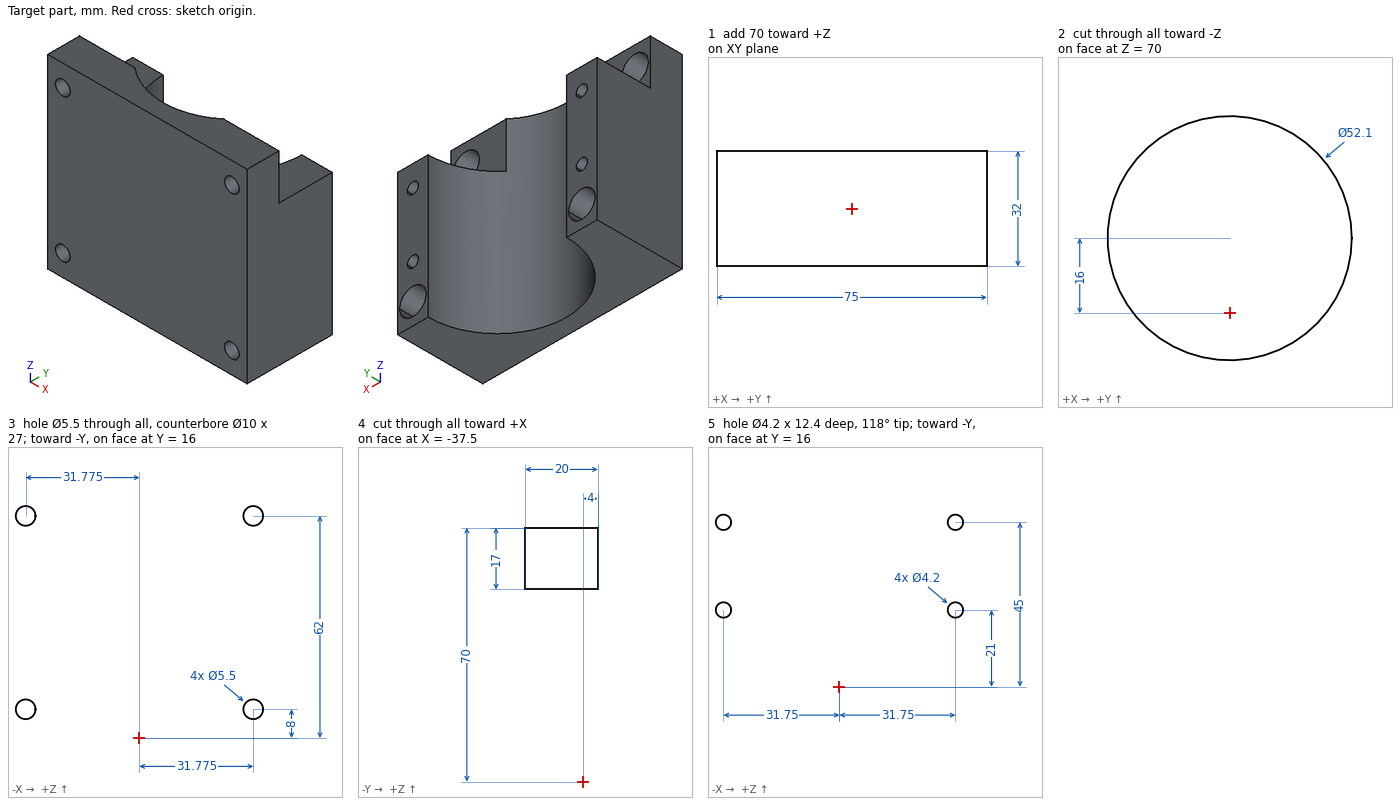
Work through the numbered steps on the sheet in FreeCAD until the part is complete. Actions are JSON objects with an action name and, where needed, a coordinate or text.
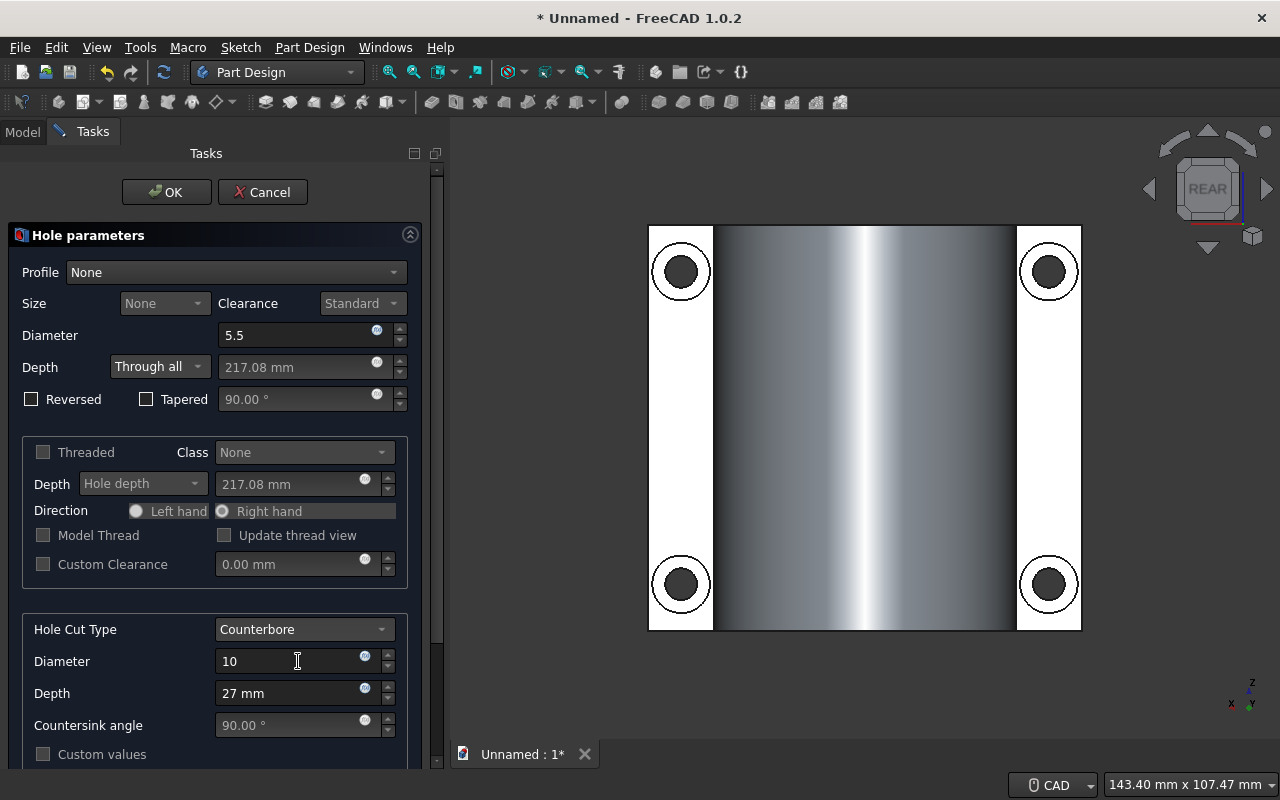
{"action": "left_click", "coordinate": [167, 192]}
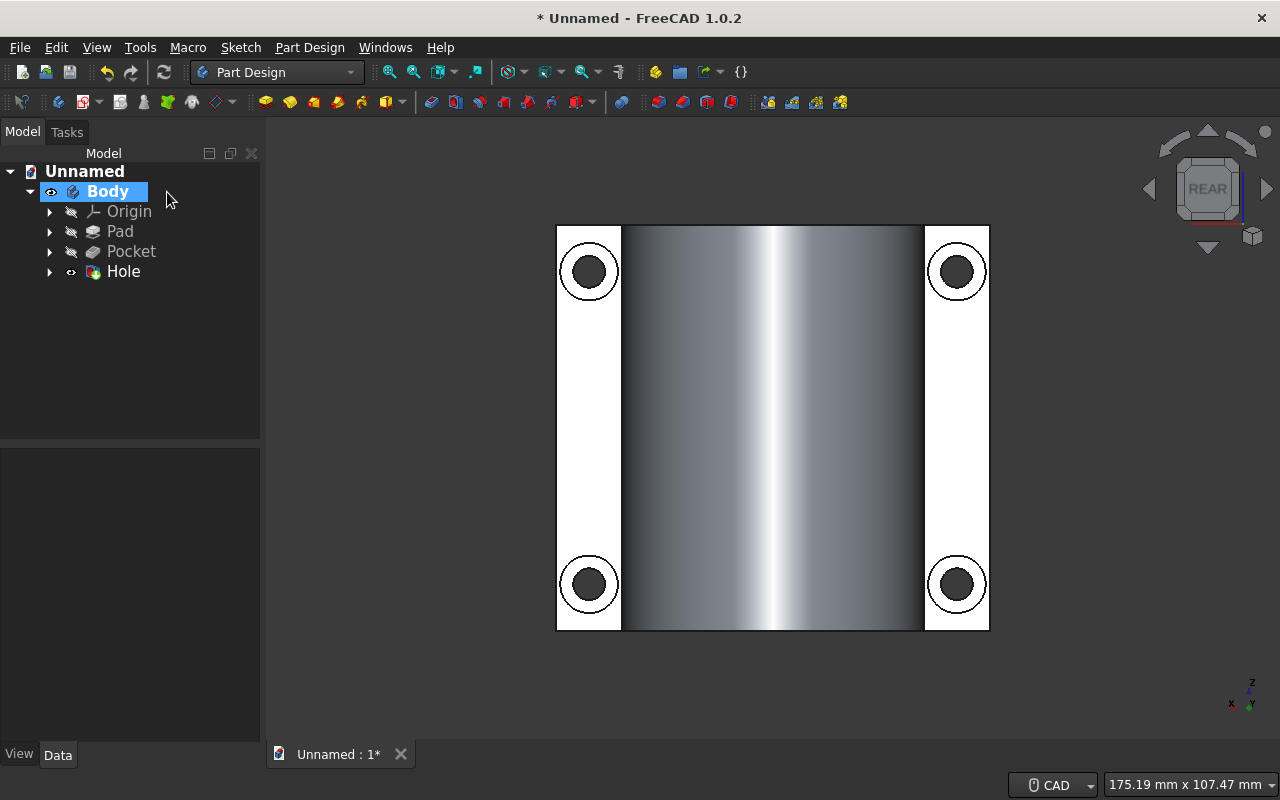
{"action": "key", "text": "6"}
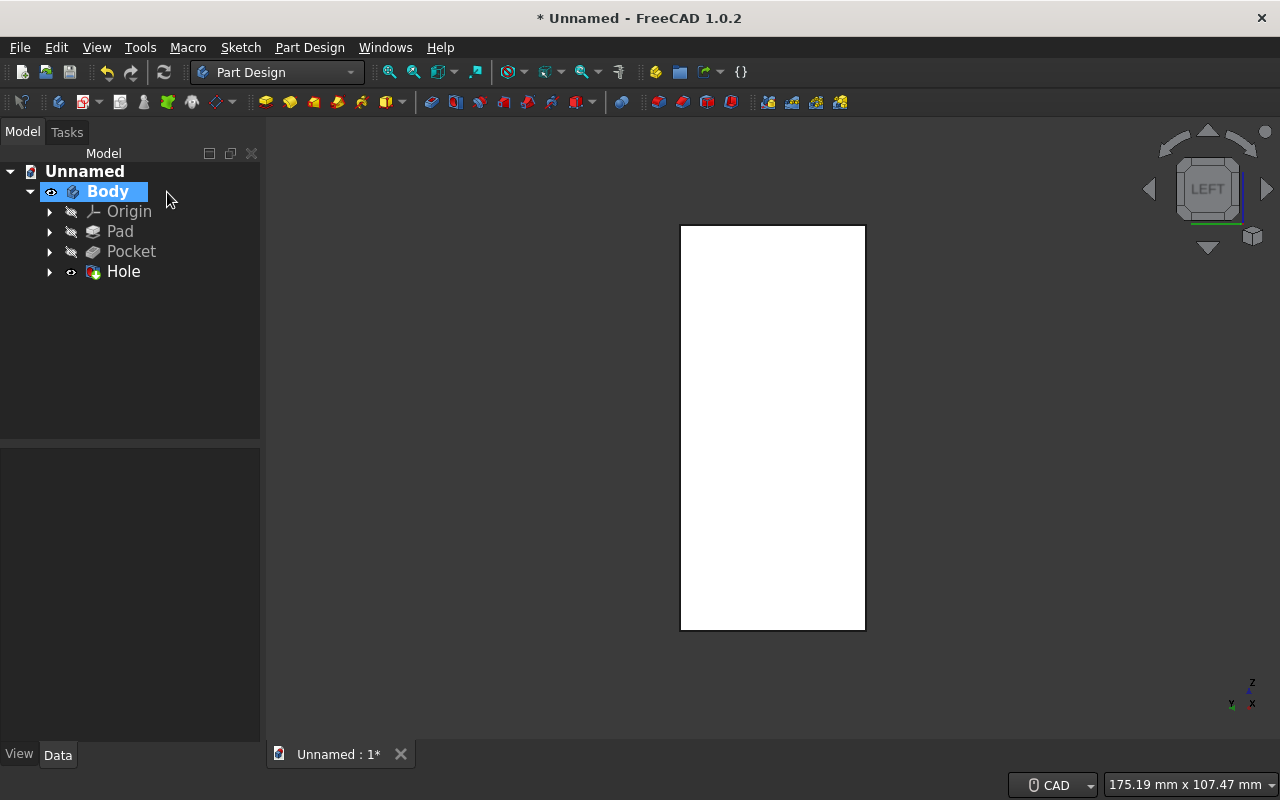
{"action": "left_click", "coordinate": [773, 369]}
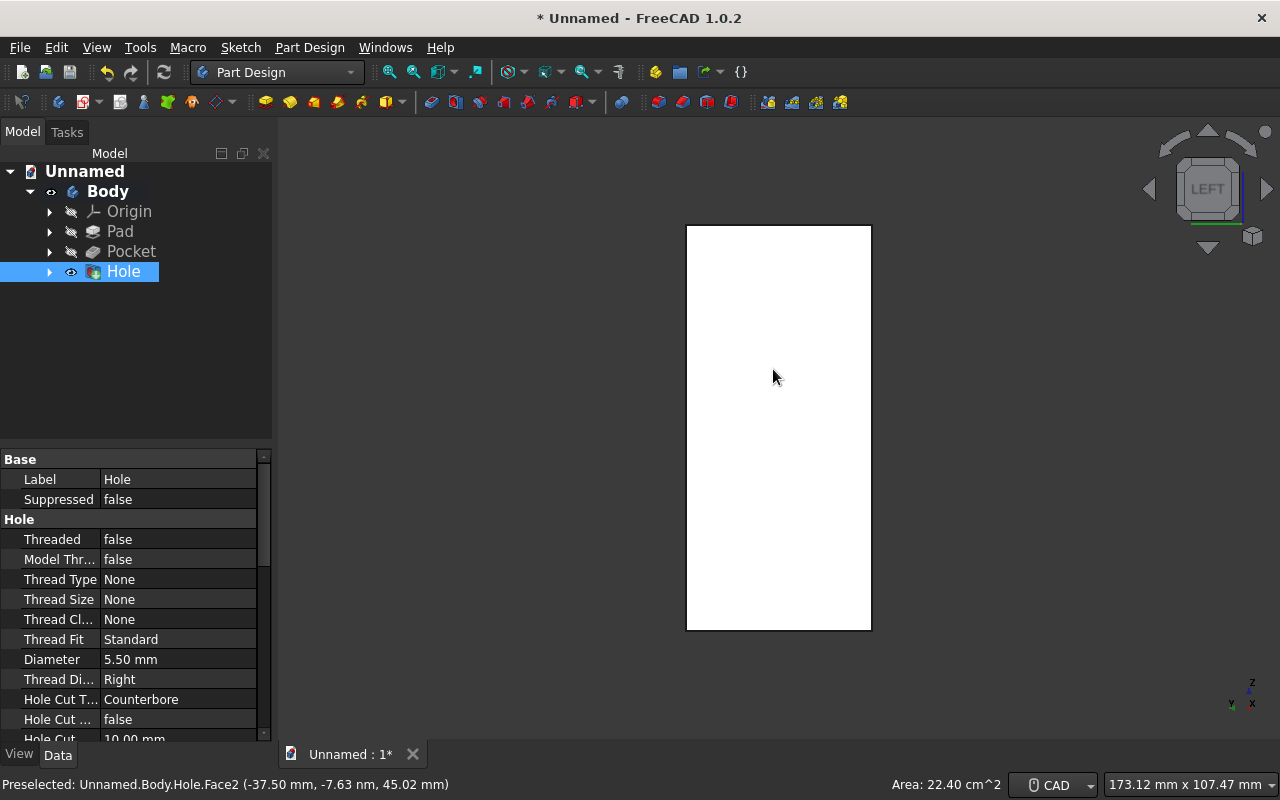
{"action": "left_click", "coordinate": [84, 102]}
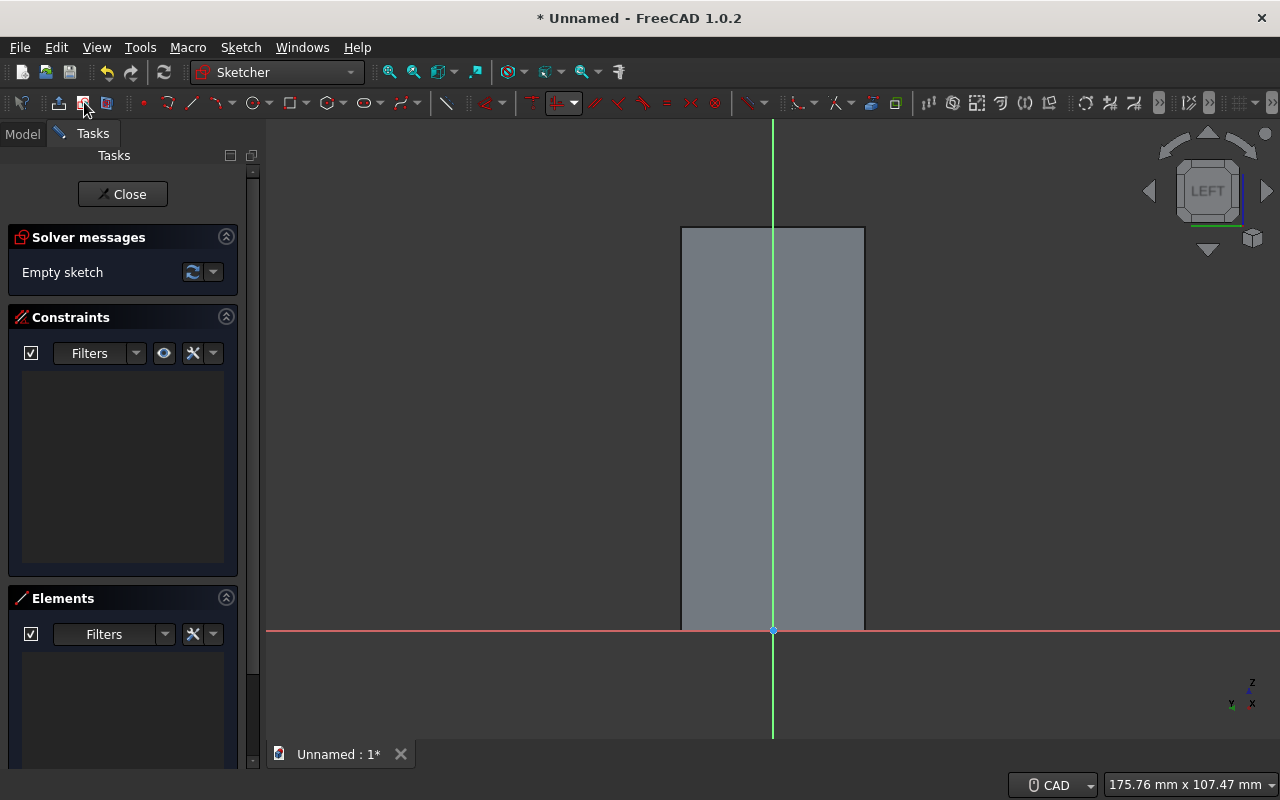
{"action": "scroll", "coordinate": [749, 226], "scroll_direction": "up", "scroll_amount": 7}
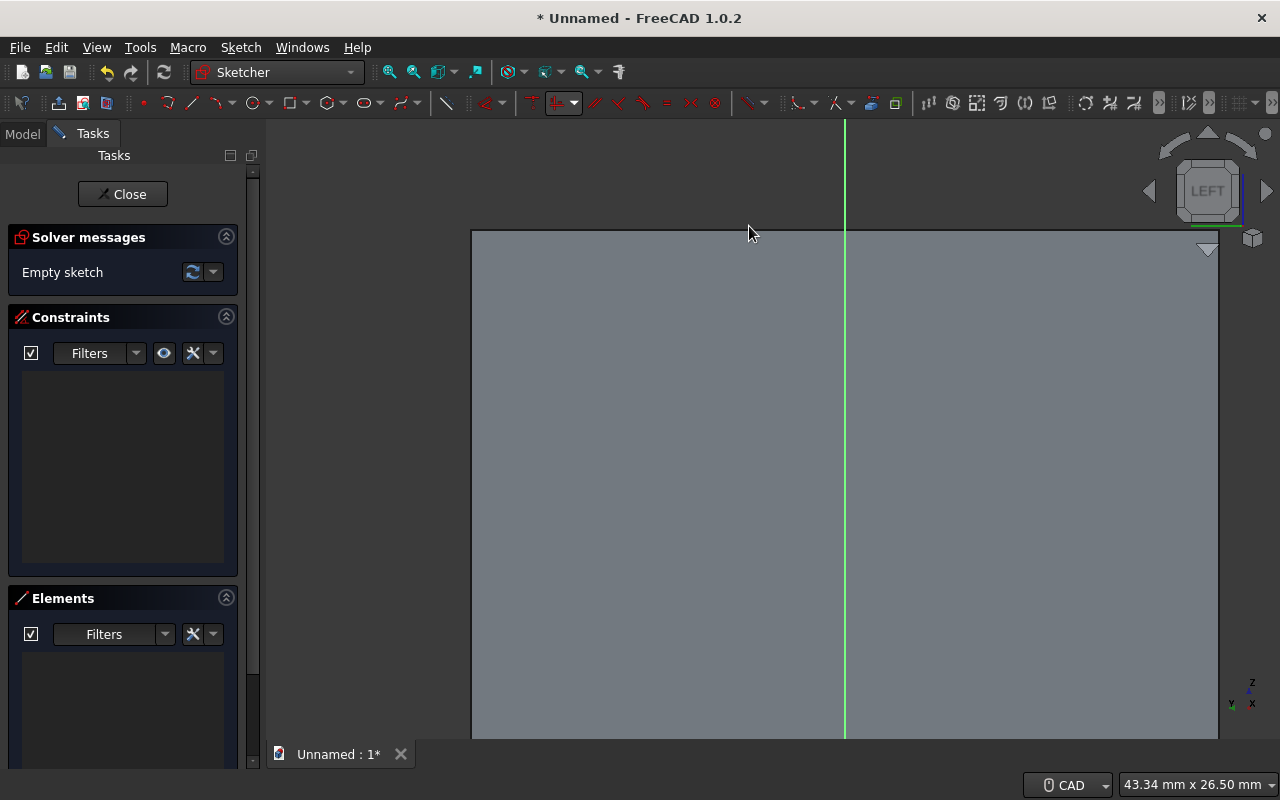
{"action": "left_click", "coordinate": [290, 104]}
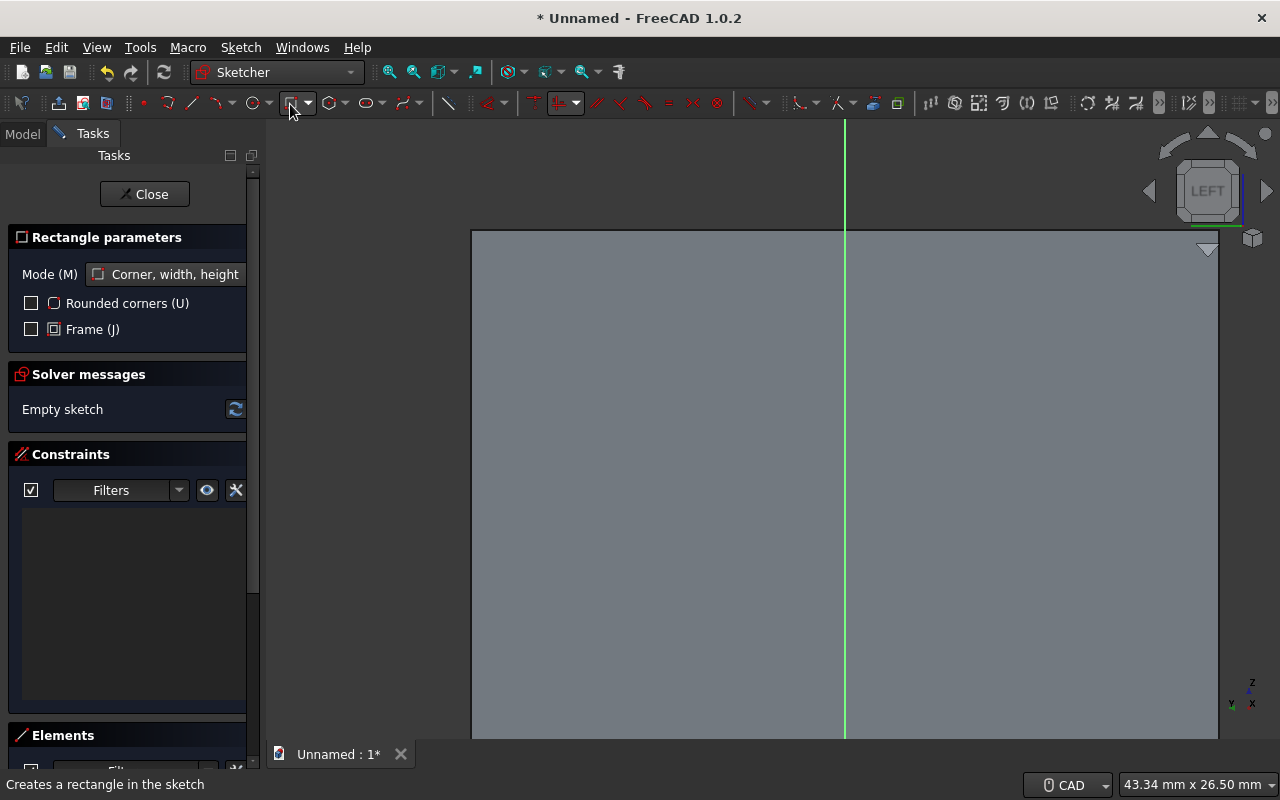
{"action": "left_click", "coordinate": [471, 230]}
{"action": "left_click", "coordinate": [938, 628]}
{"action": "key", "text": "Escape"}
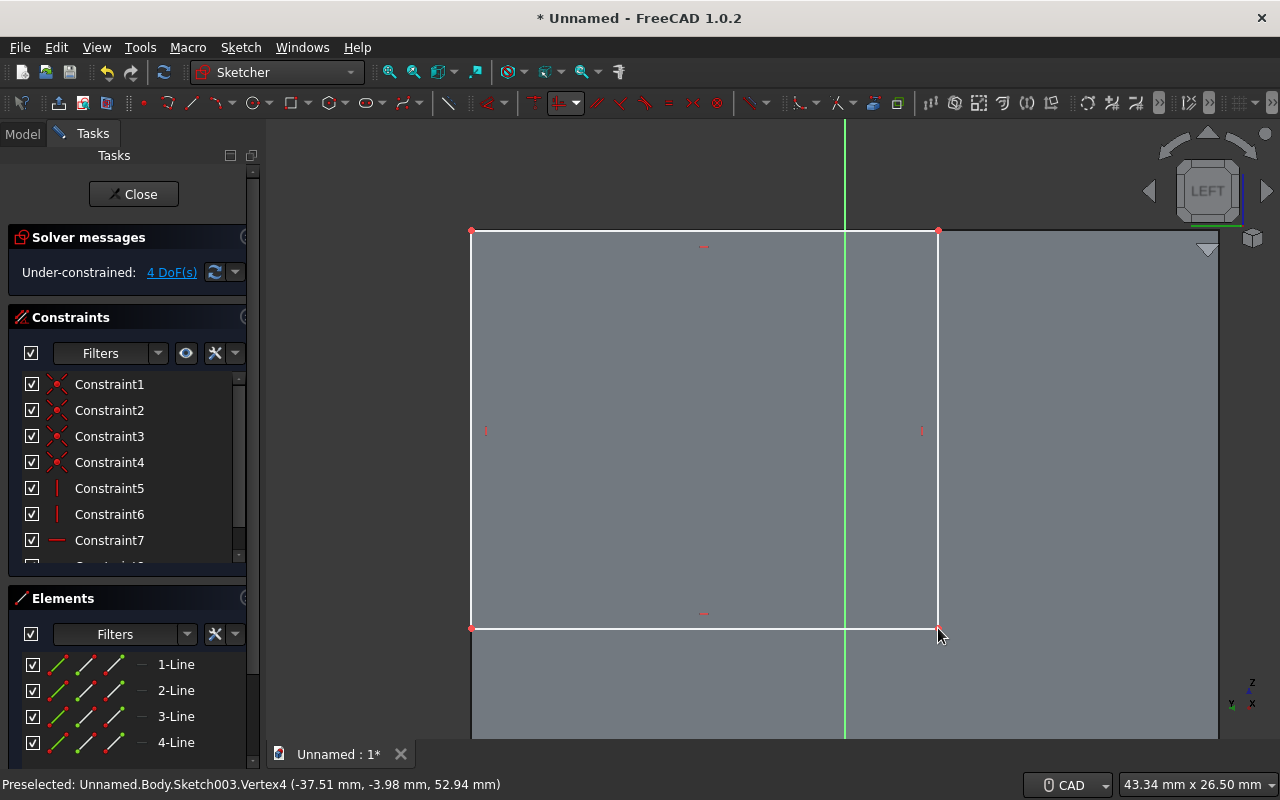
{"action": "left_click", "coordinate": [488, 104]}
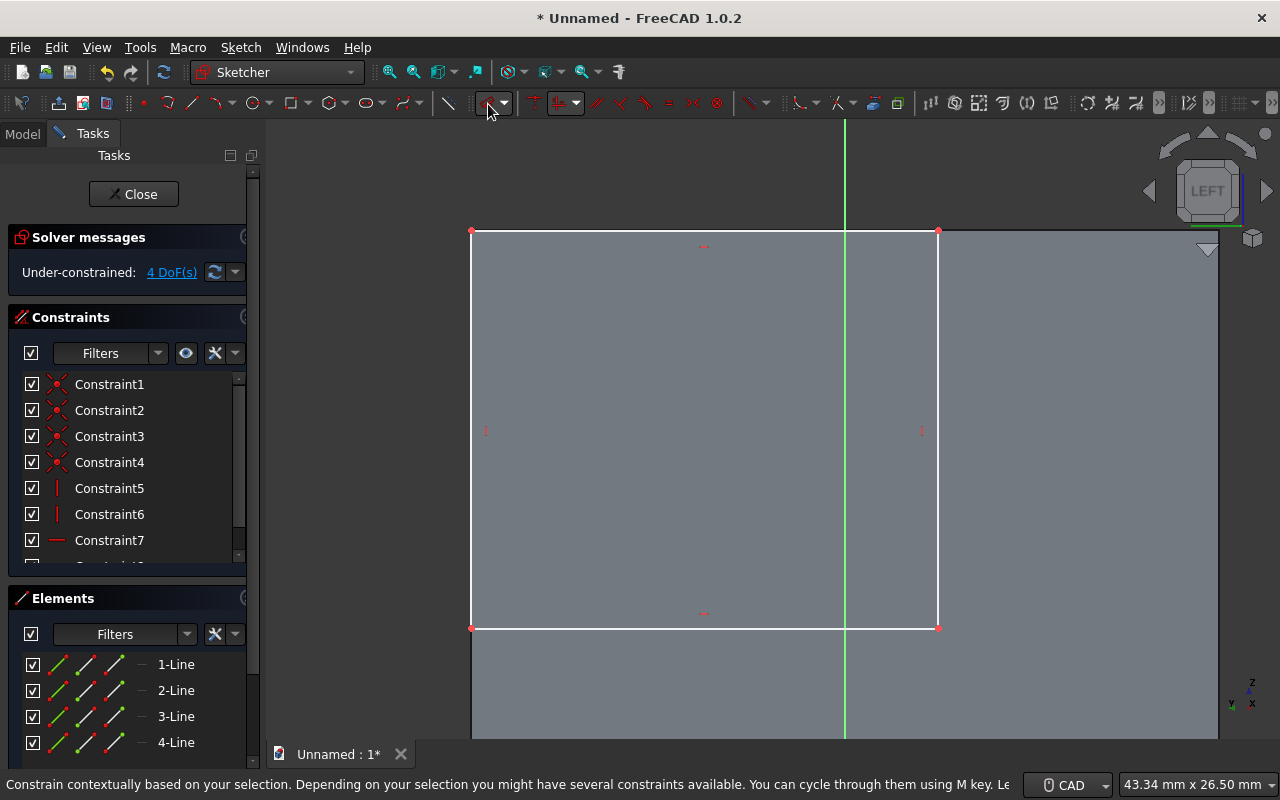
{"action": "left_click", "coordinate": [471, 350]}
{"action": "left_click", "coordinate": [437, 430]}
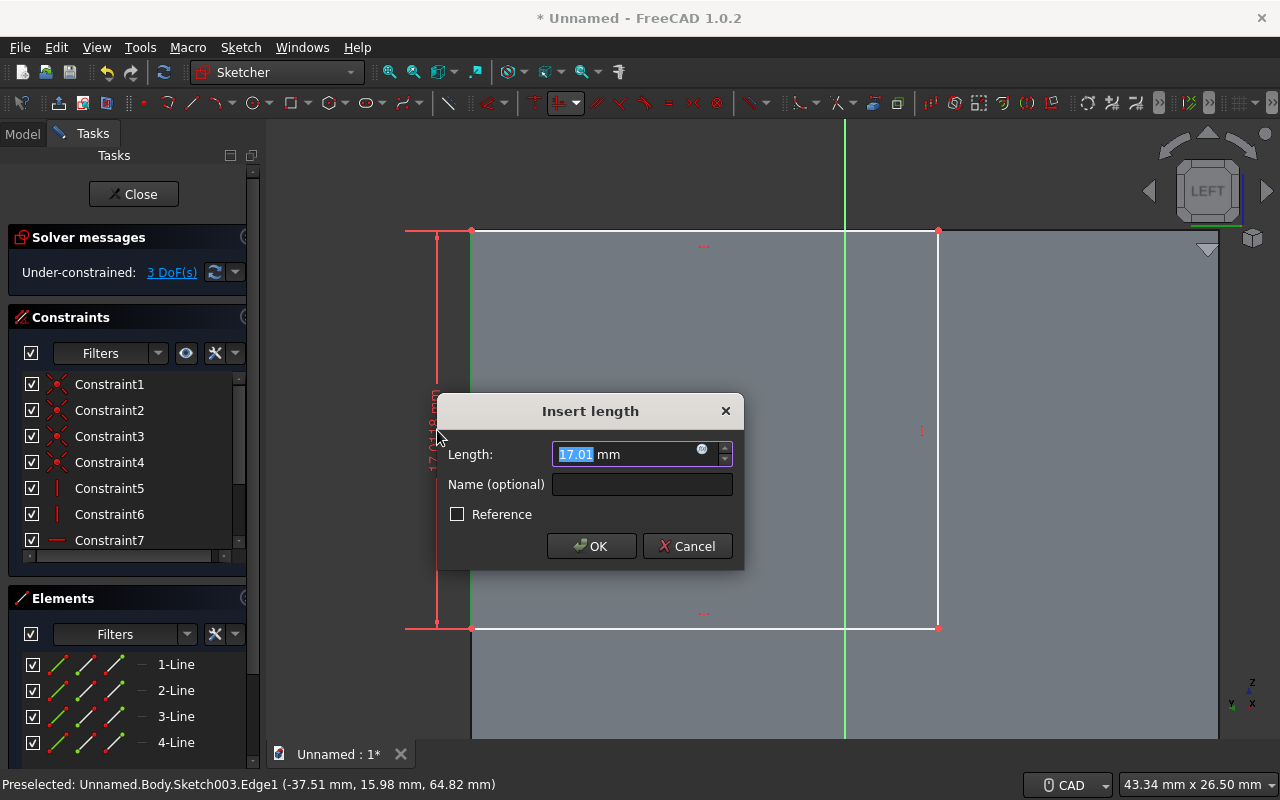
{"action": "type", "text": "17"}
{"action": "key", "text": "Return"}